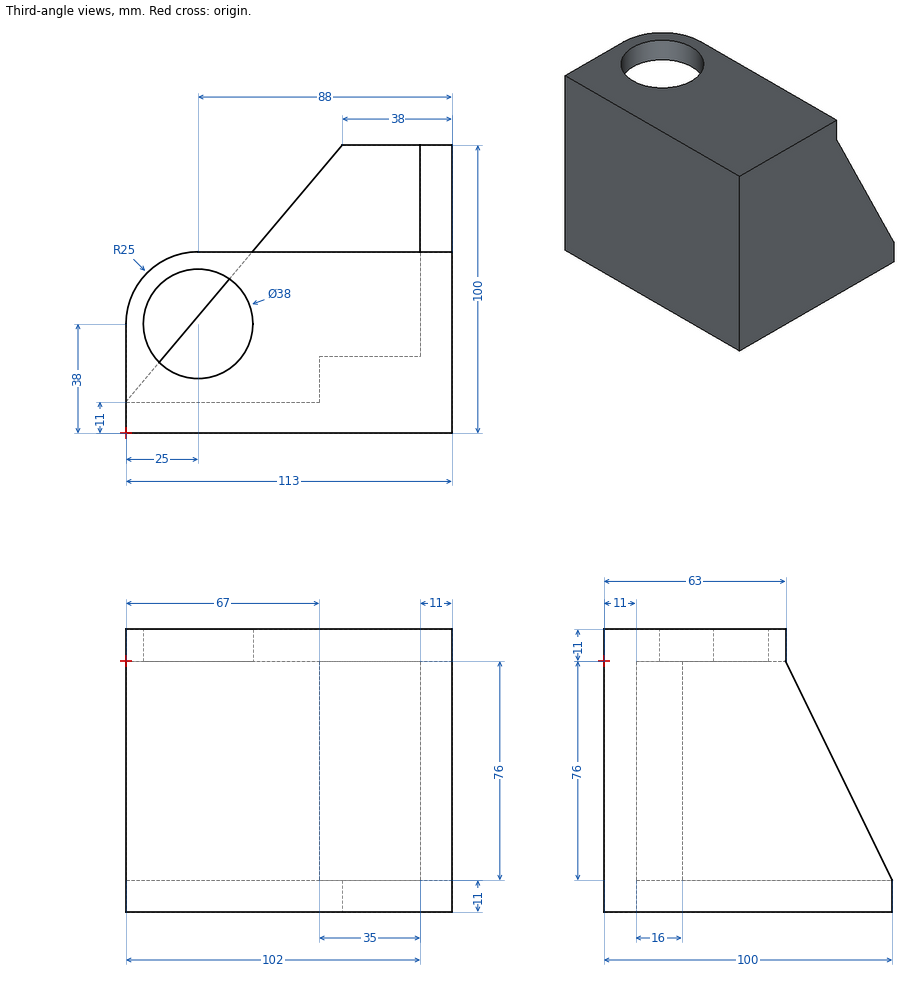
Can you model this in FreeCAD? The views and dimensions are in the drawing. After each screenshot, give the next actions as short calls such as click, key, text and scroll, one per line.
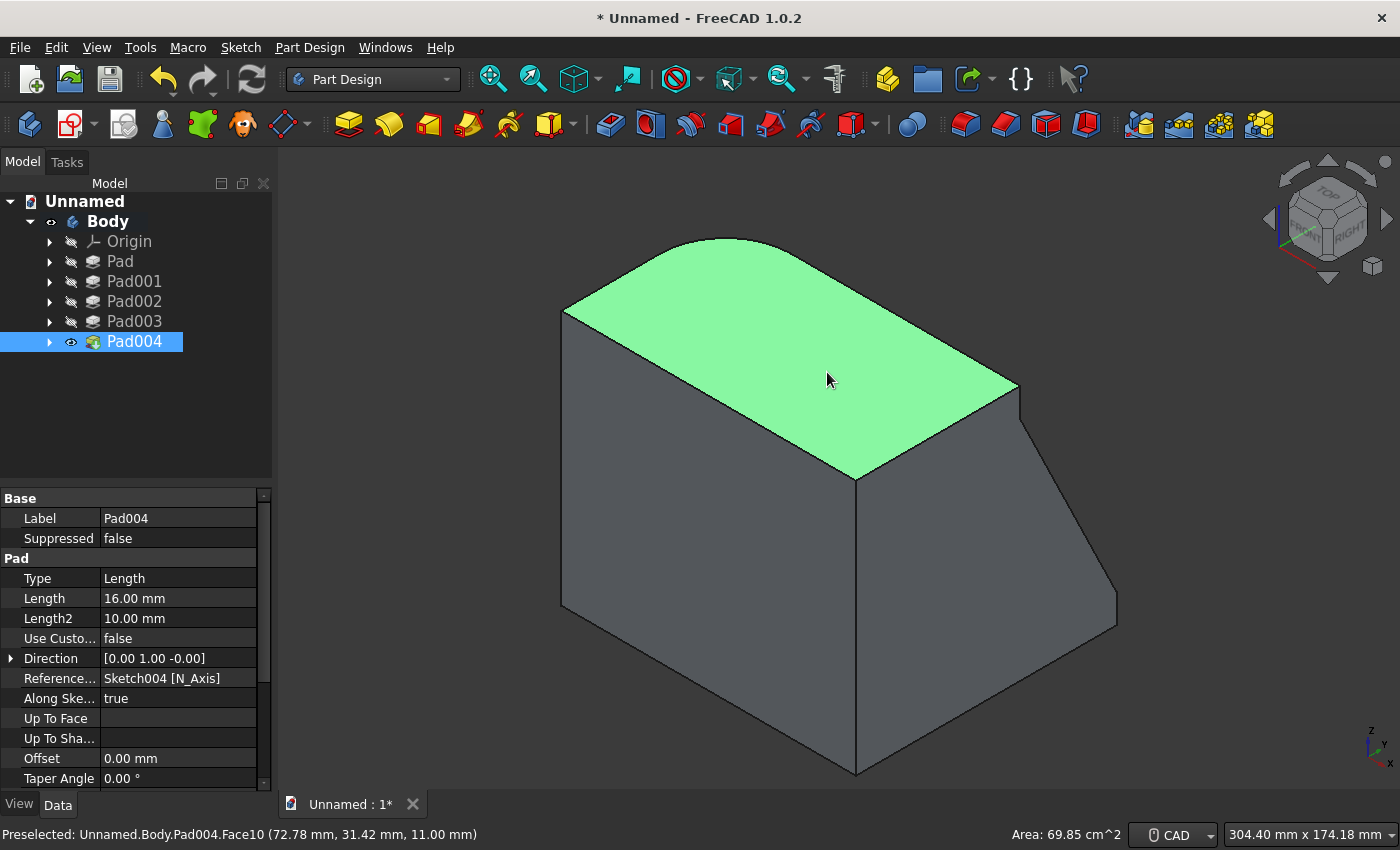
click(70, 124)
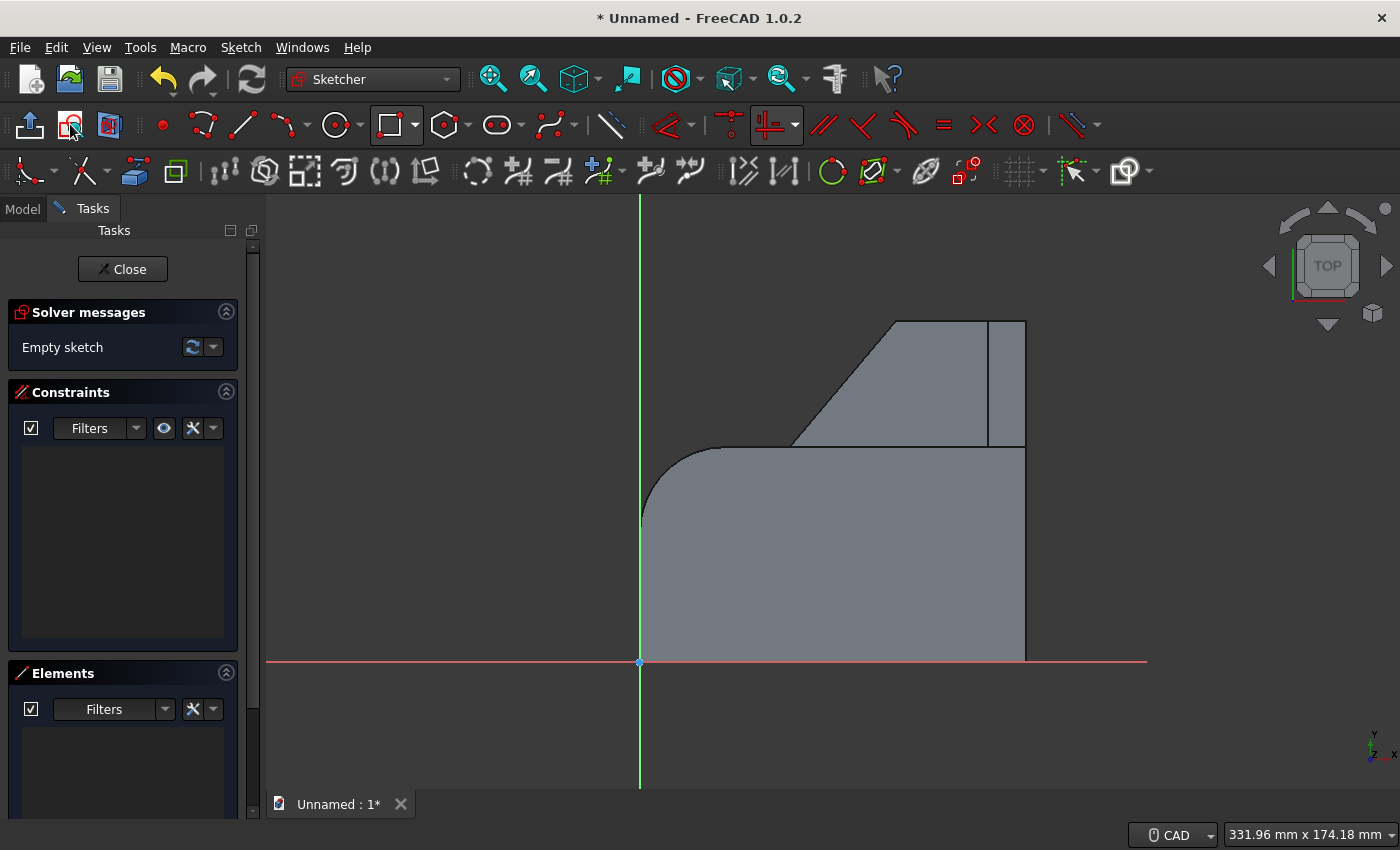
scroll(655, 654, up, 3)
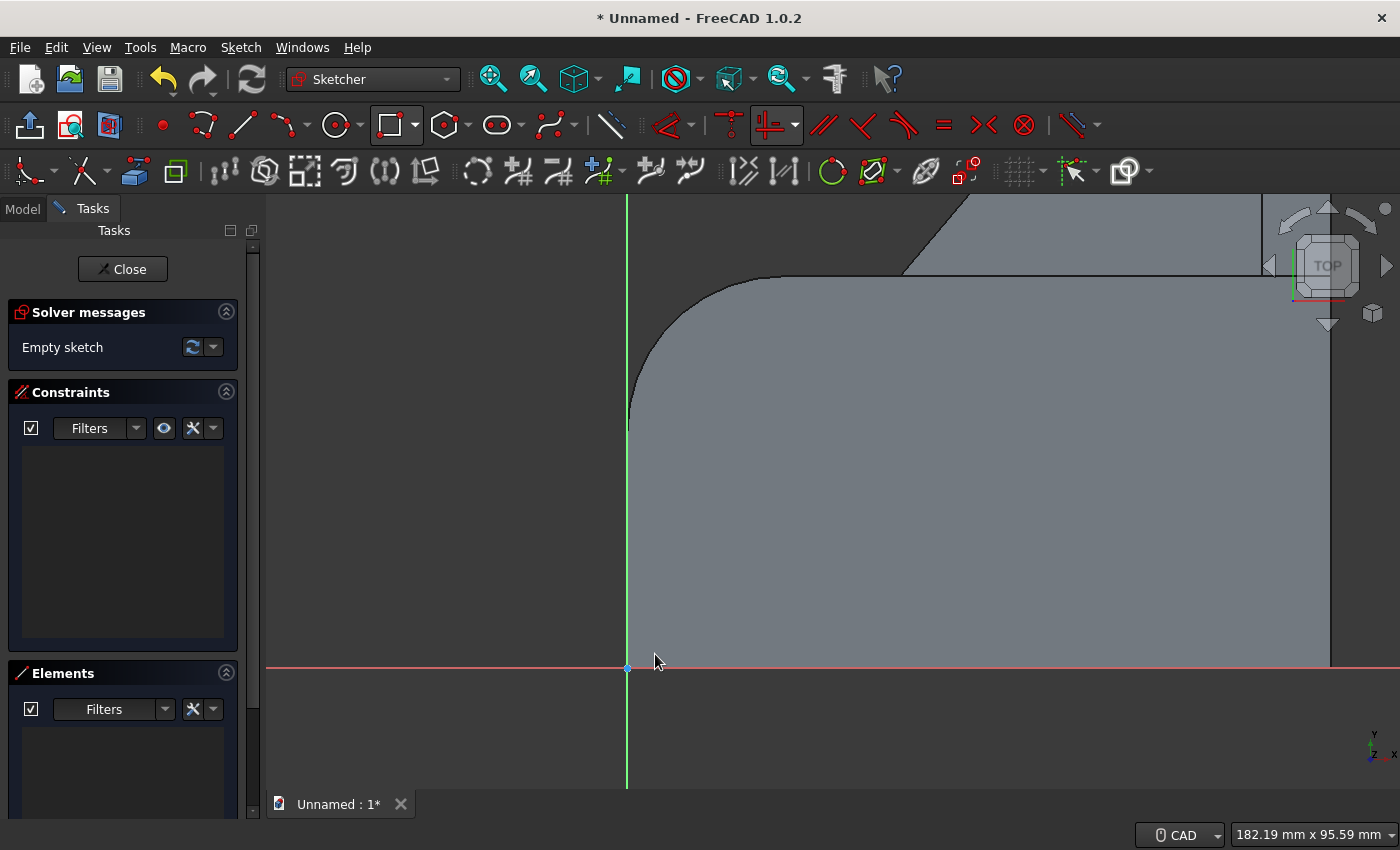
key(g)
key(c)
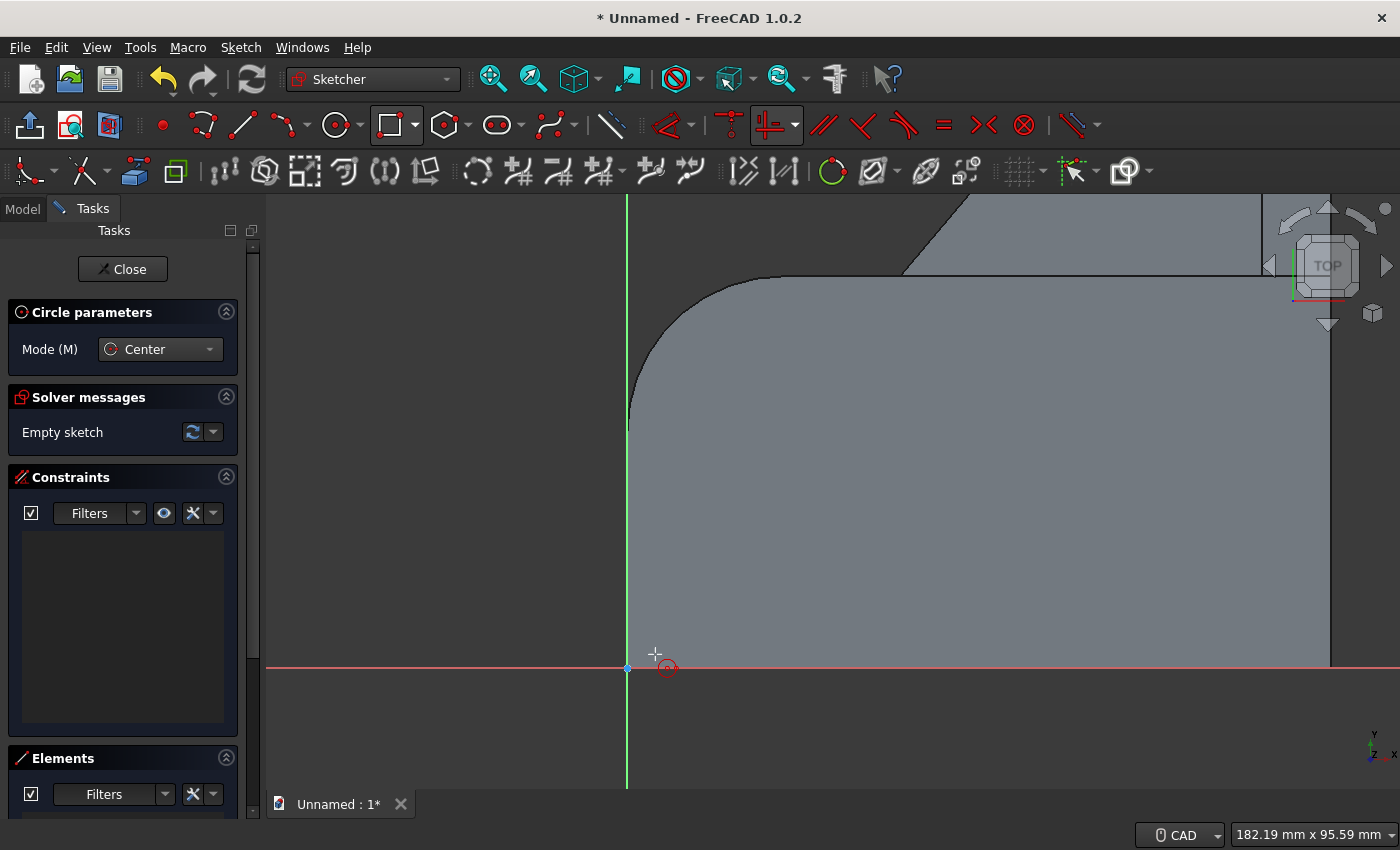
click(783, 432)
move(867, 348)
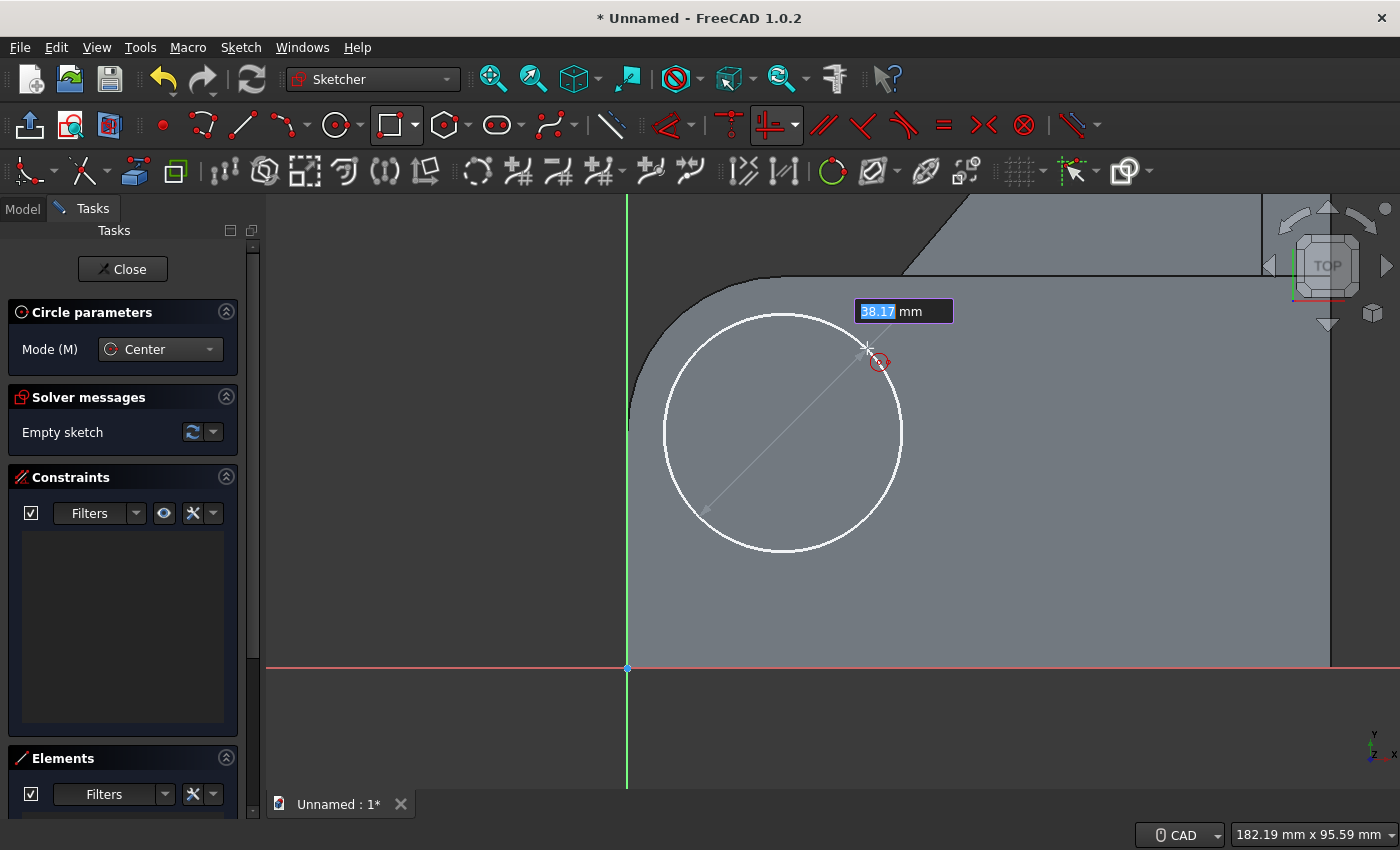
text(38)
key(Return)
key(Escape)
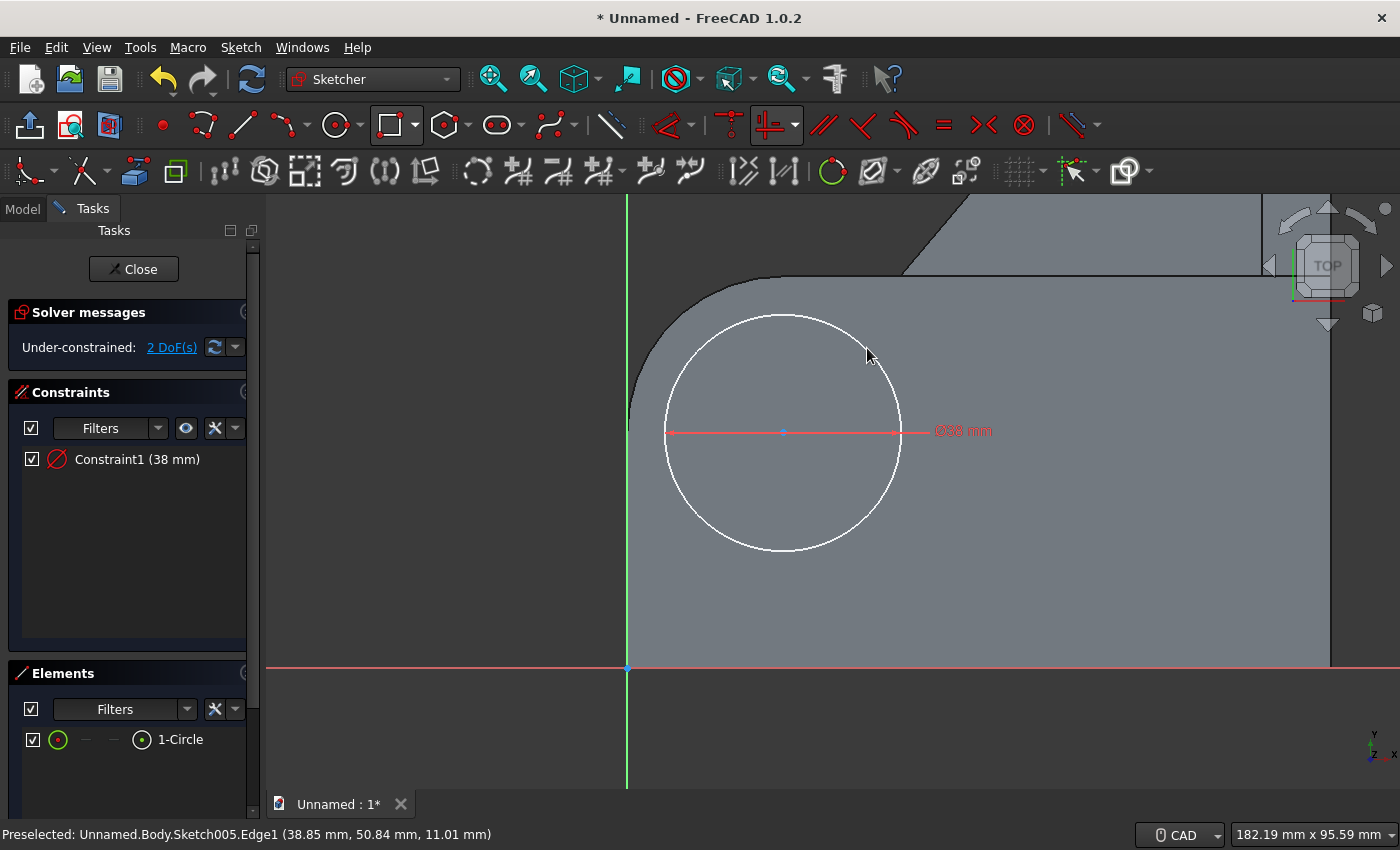
click(666, 126)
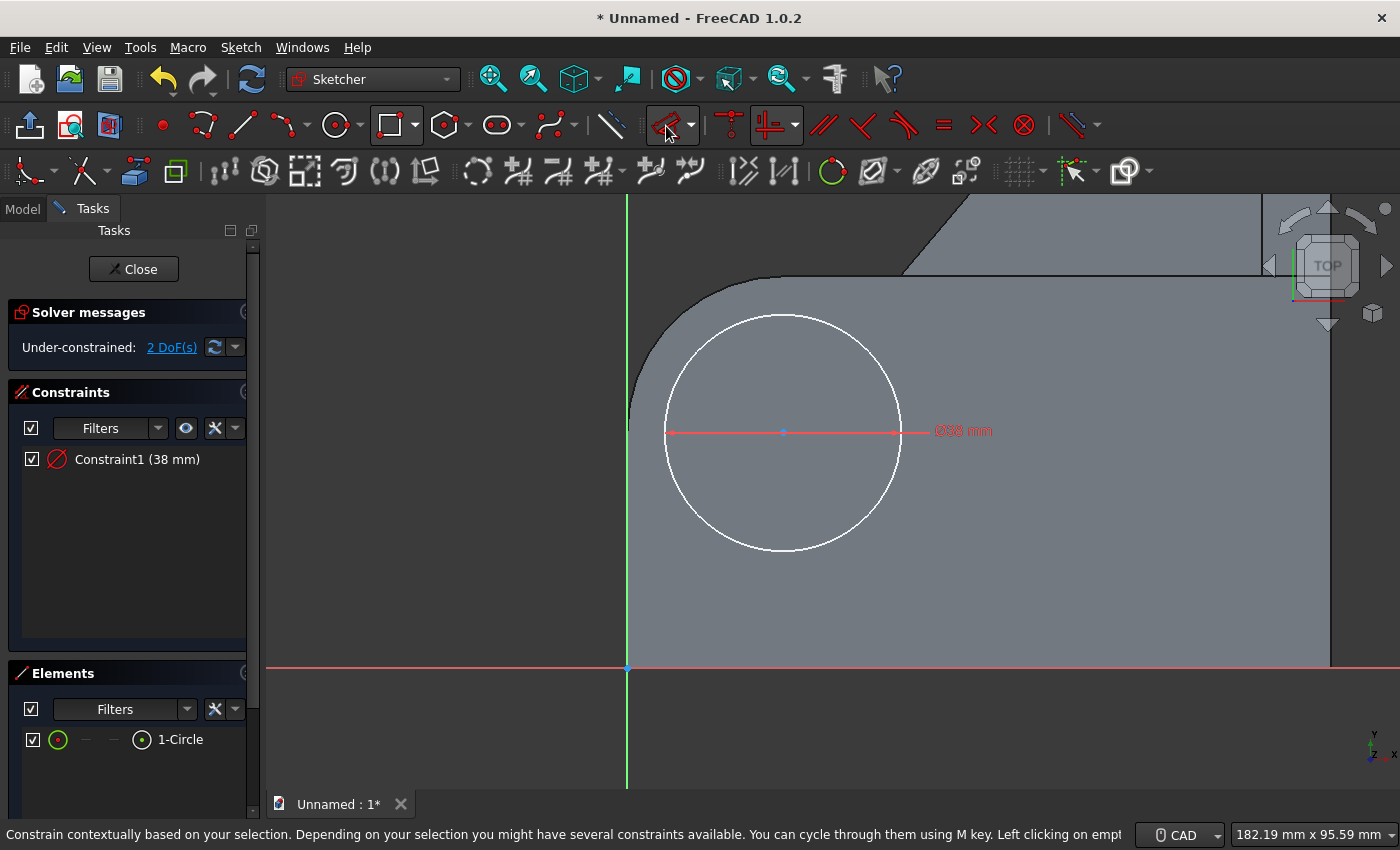
click(783, 433)
click(705, 702)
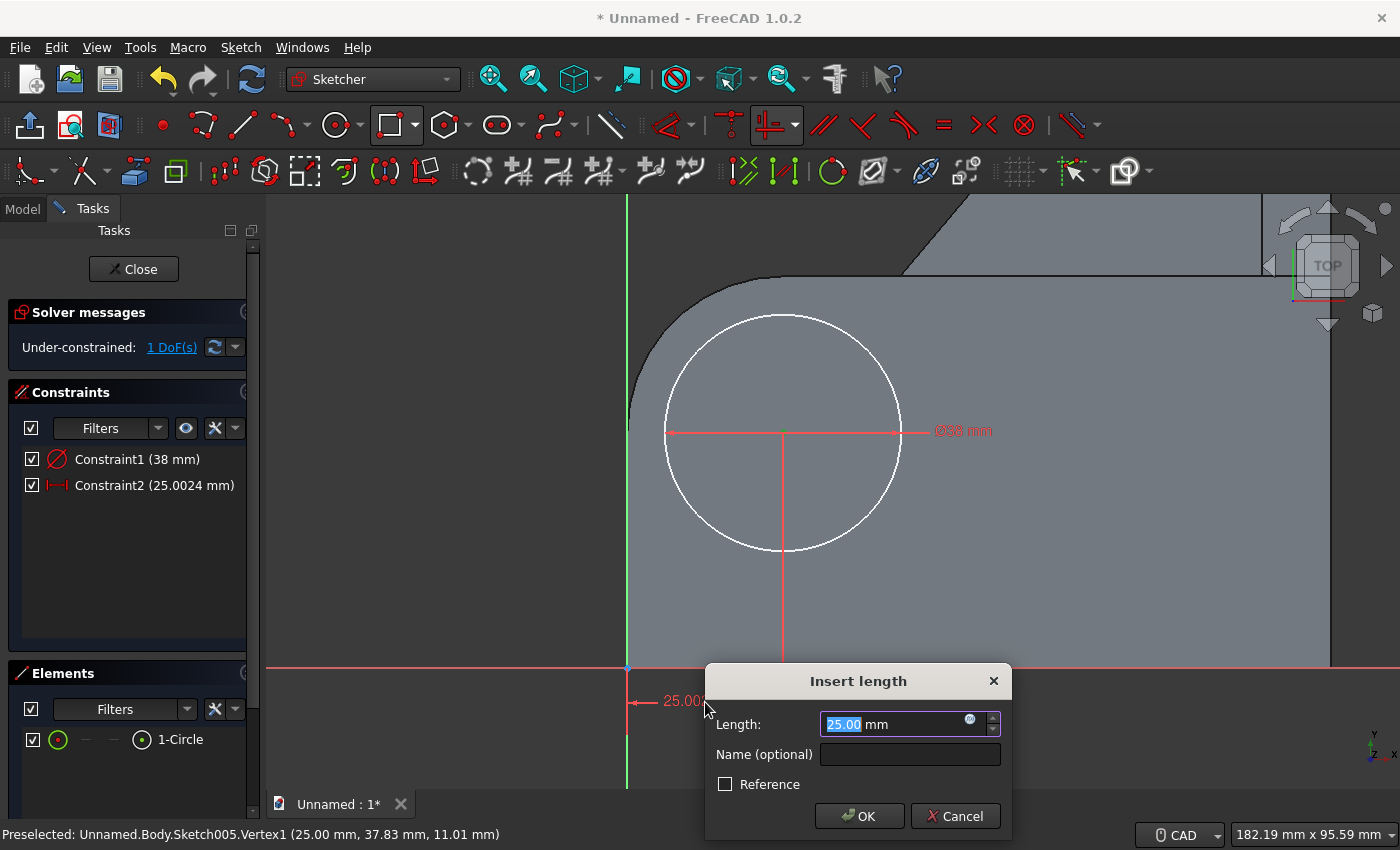
text(25)
key(Return)